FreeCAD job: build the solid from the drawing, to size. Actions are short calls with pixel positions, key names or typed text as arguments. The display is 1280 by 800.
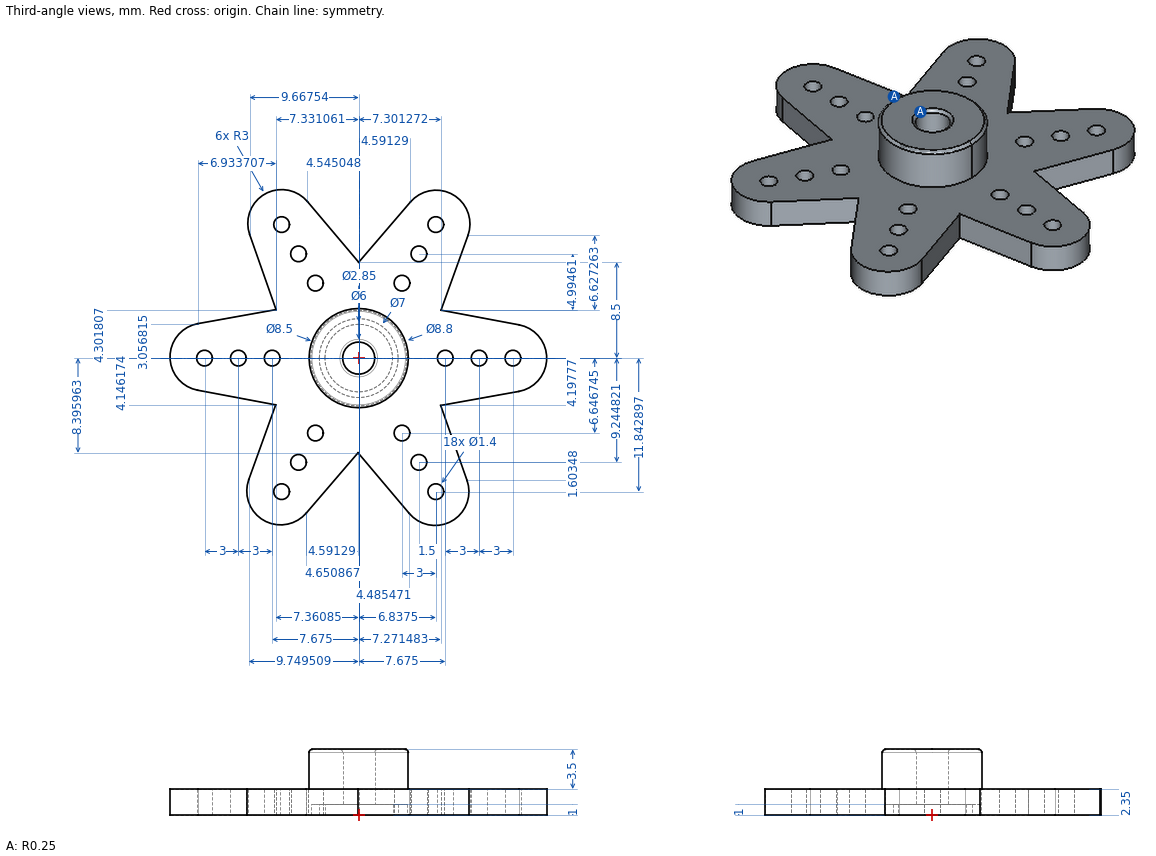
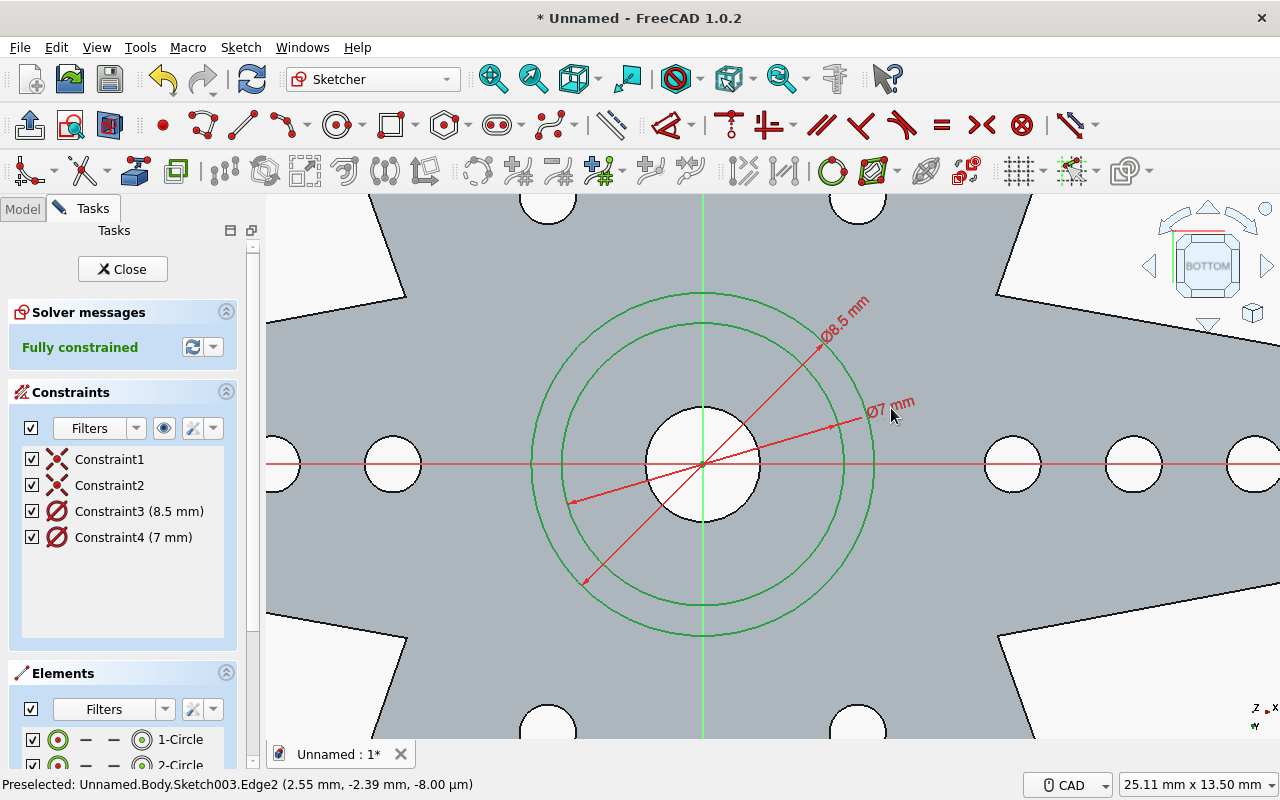
click(123, 269)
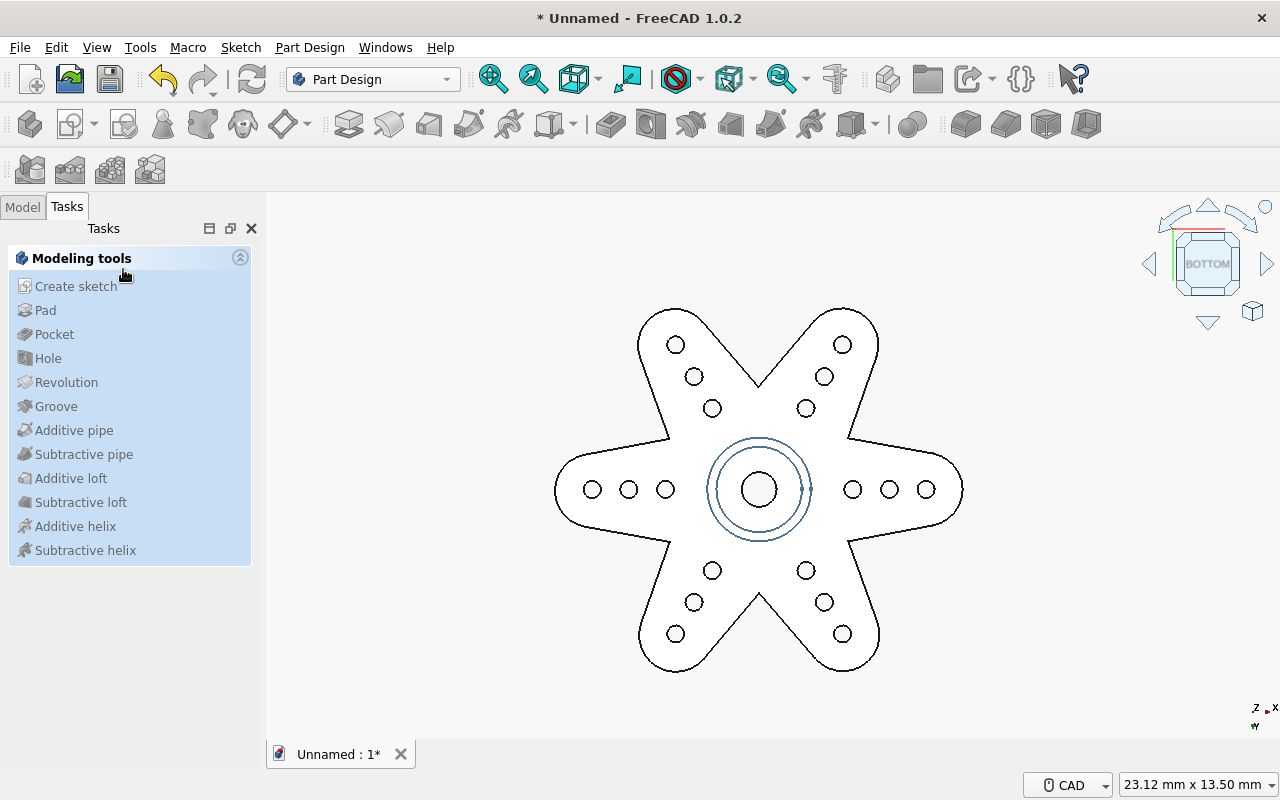
click(612, 124)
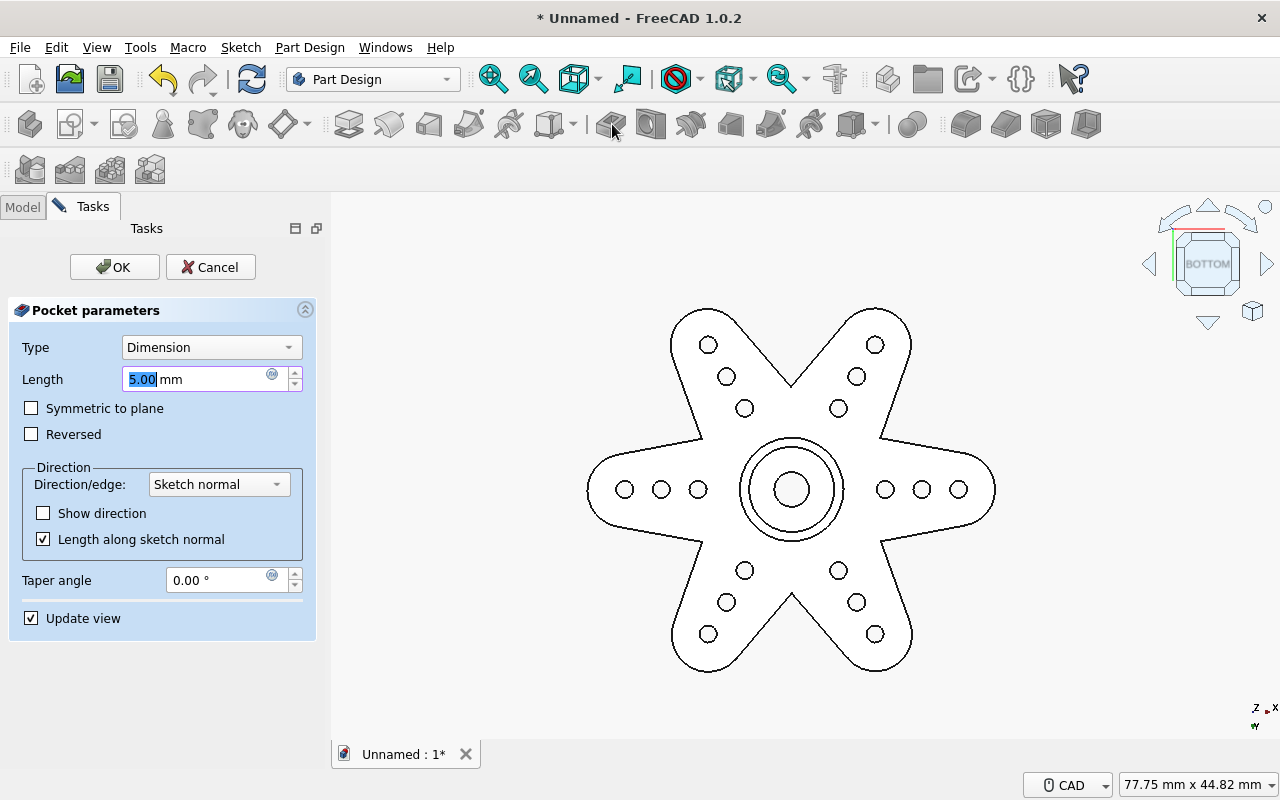
text(1)
key(Tab)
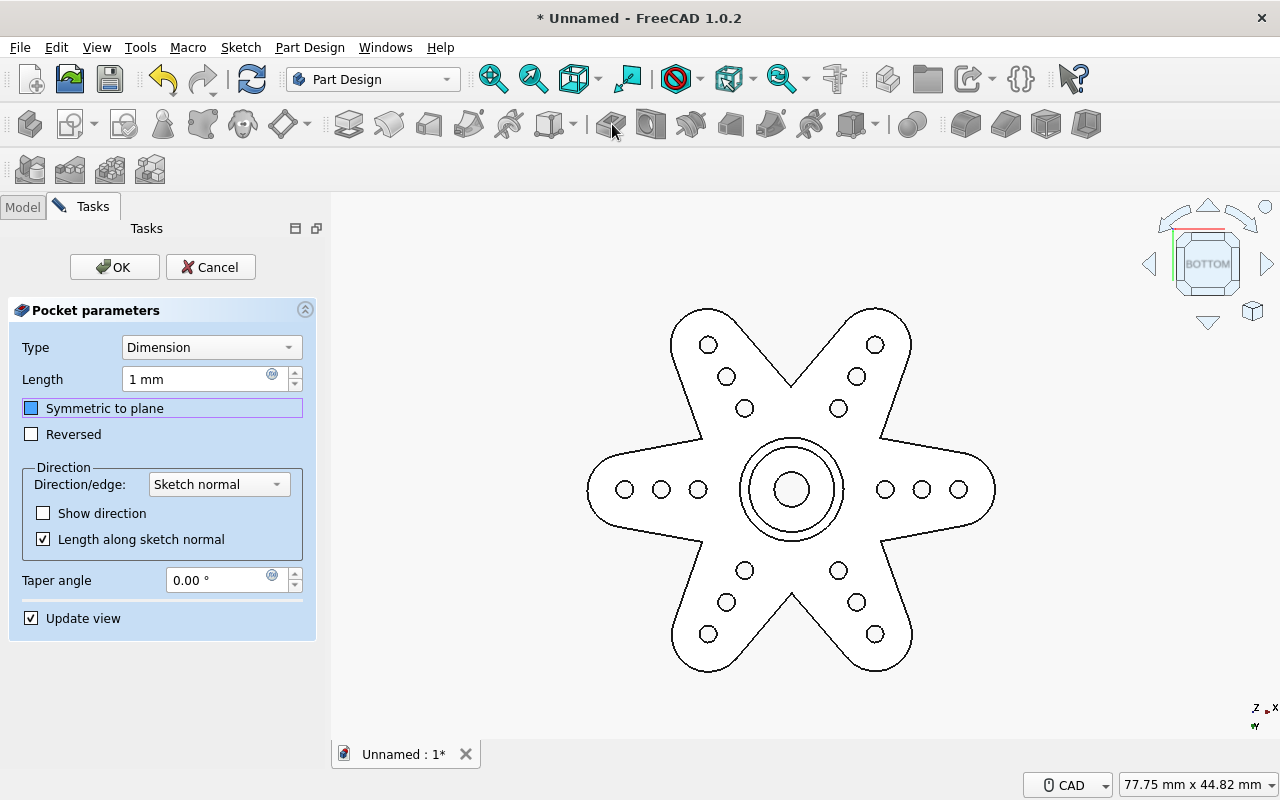
click(115, 267)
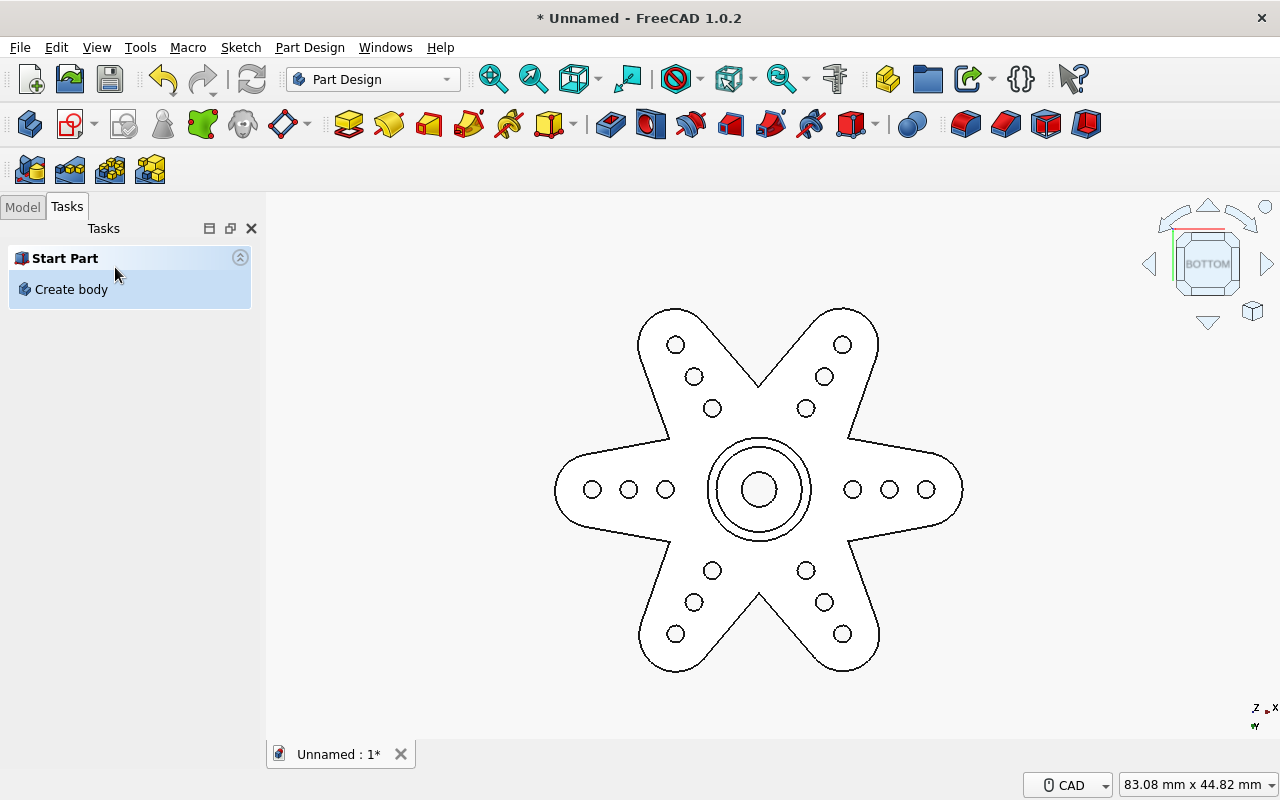
click(70, 124)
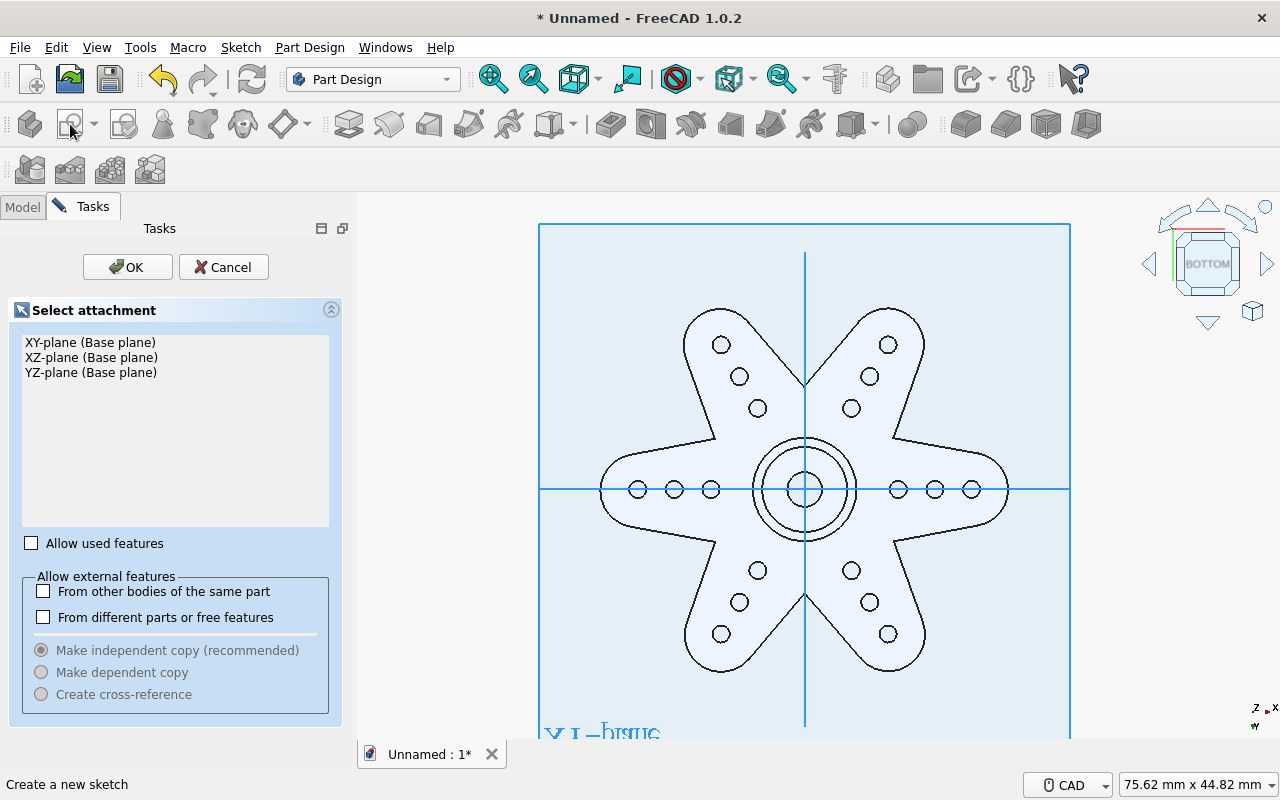
click(82, 342)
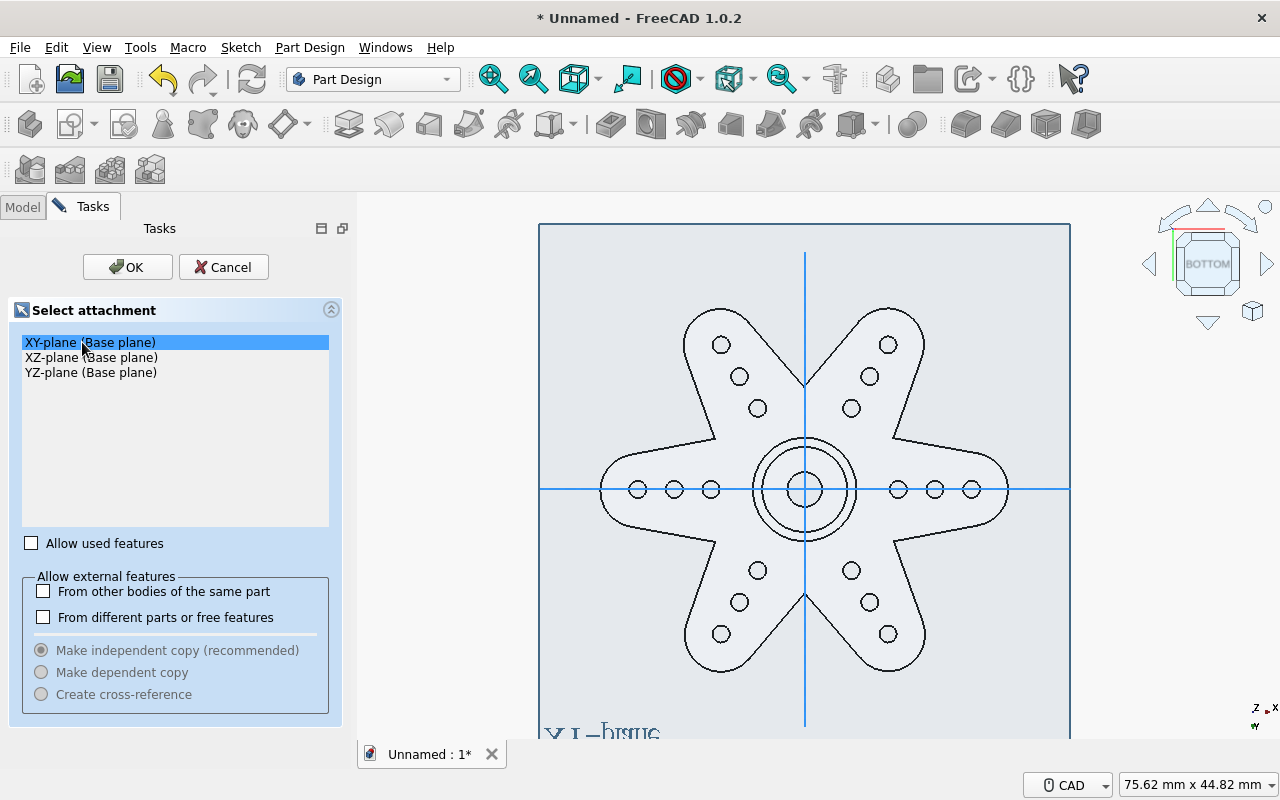
click(128, 267)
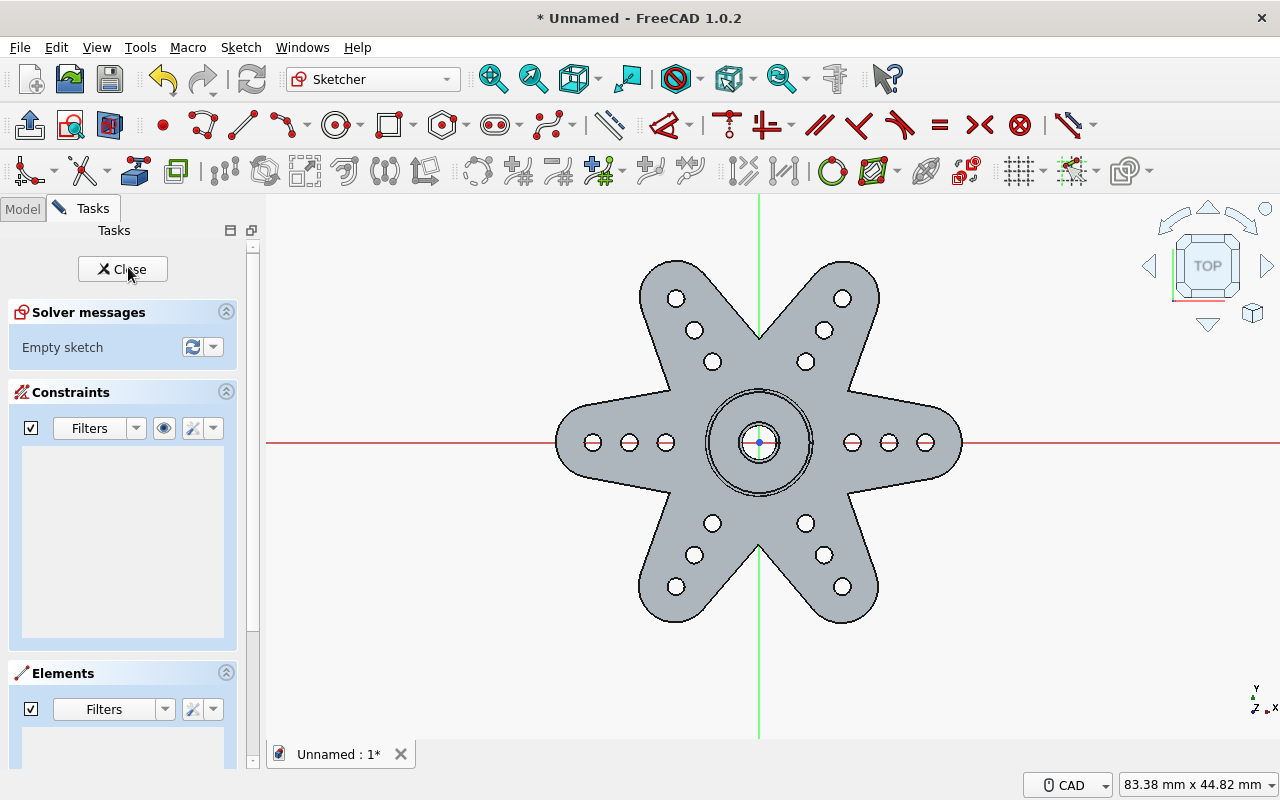
click(110, 126)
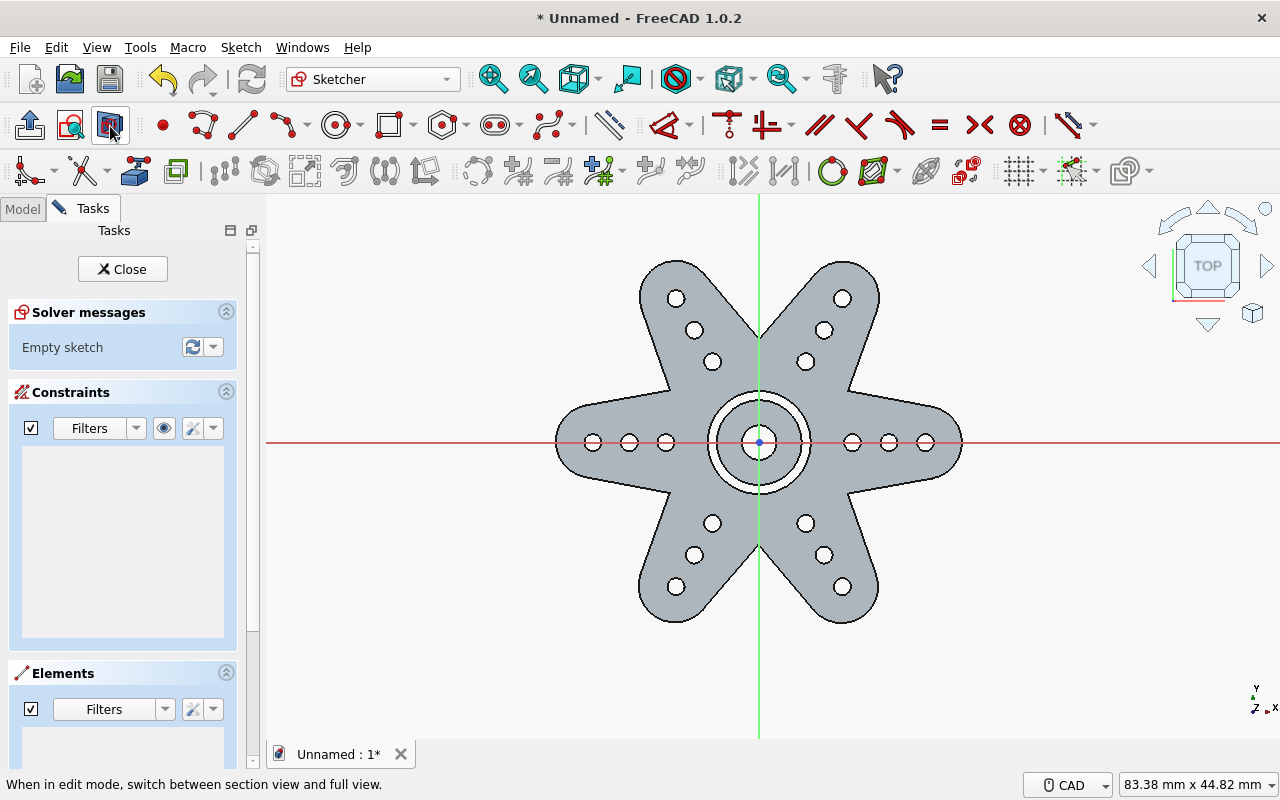
scroll(773, 437, up, 8)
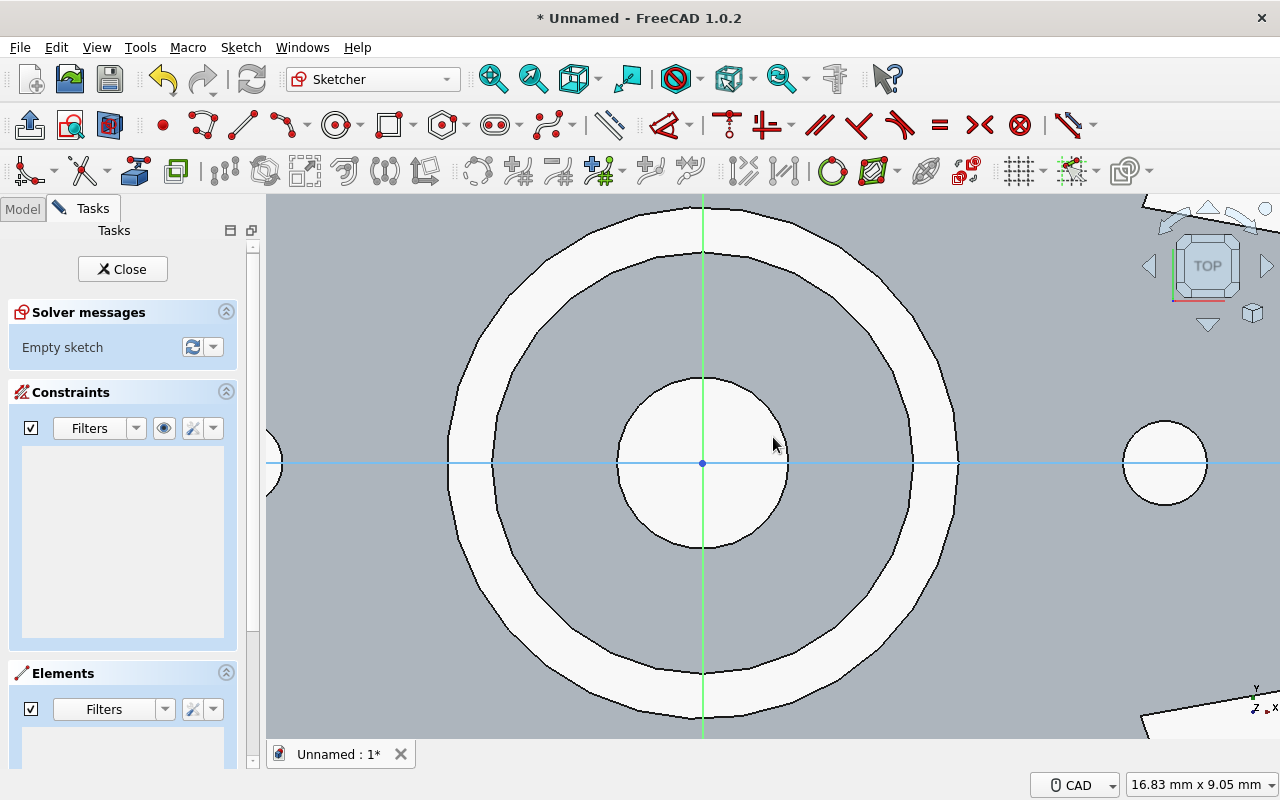
click(336, 126)